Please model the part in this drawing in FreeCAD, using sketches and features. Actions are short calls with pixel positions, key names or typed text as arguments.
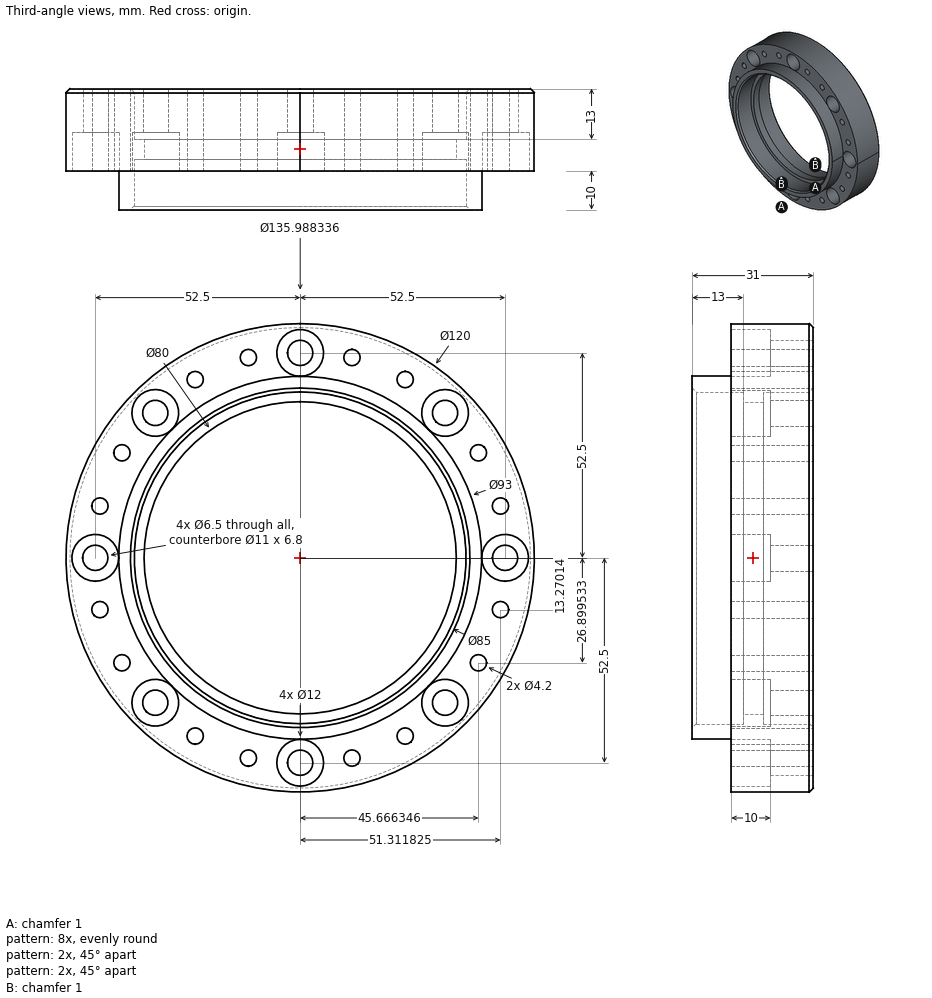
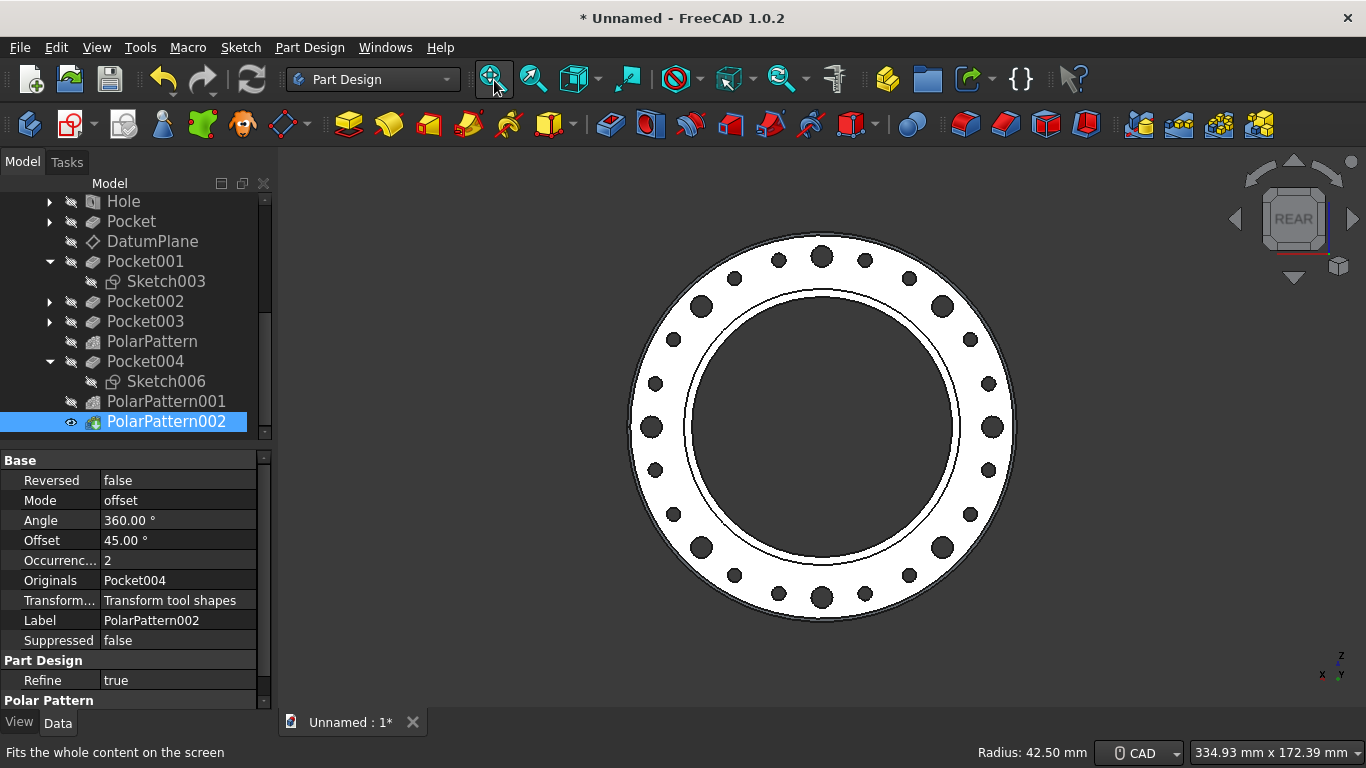
click(960, 426, ctrl)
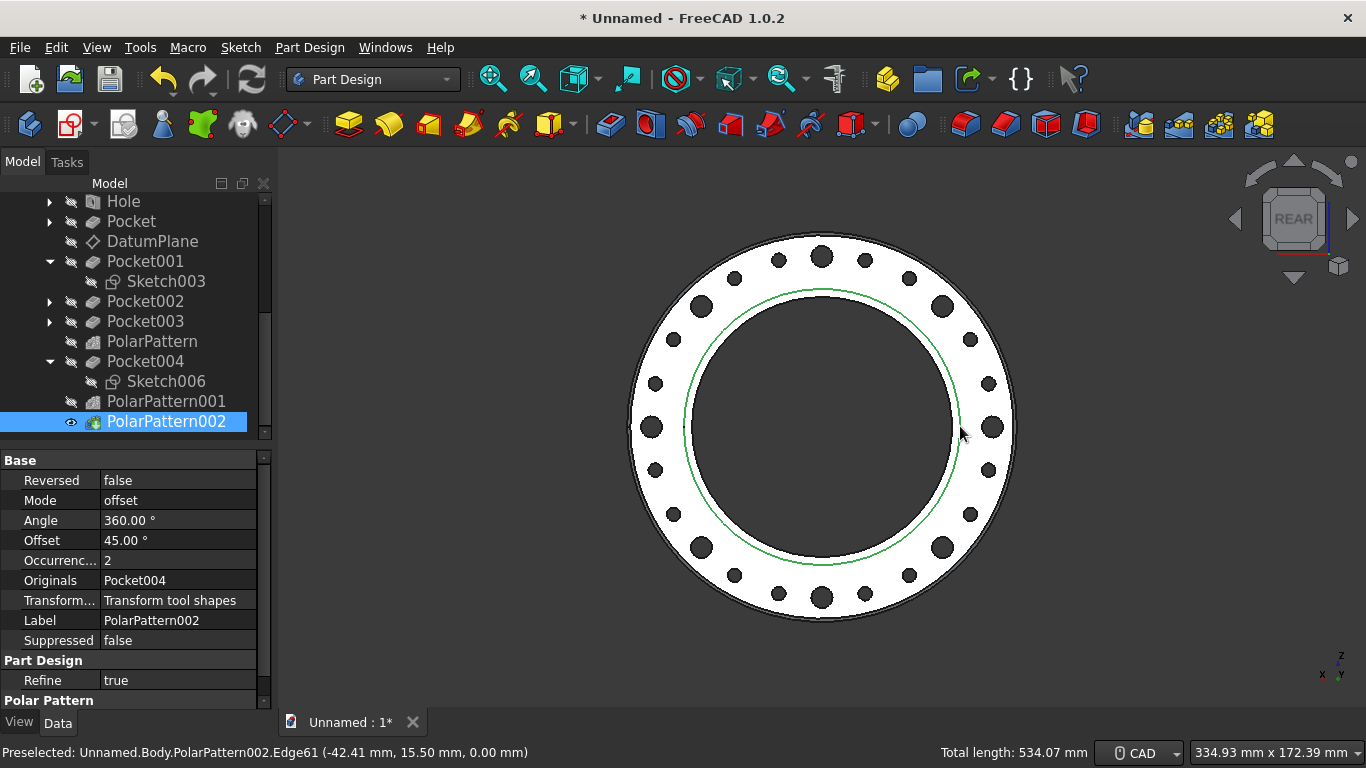
click(1006, 124)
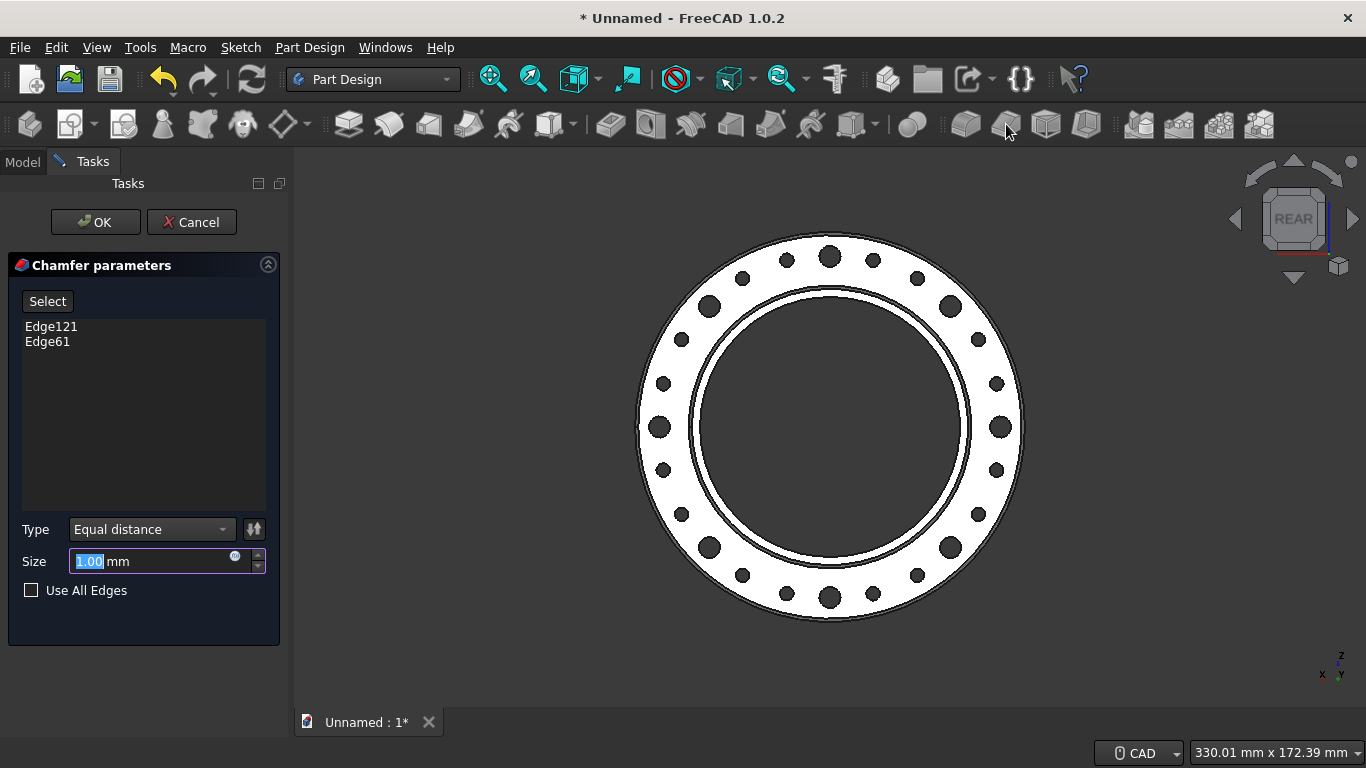
text(1)
key(Tab)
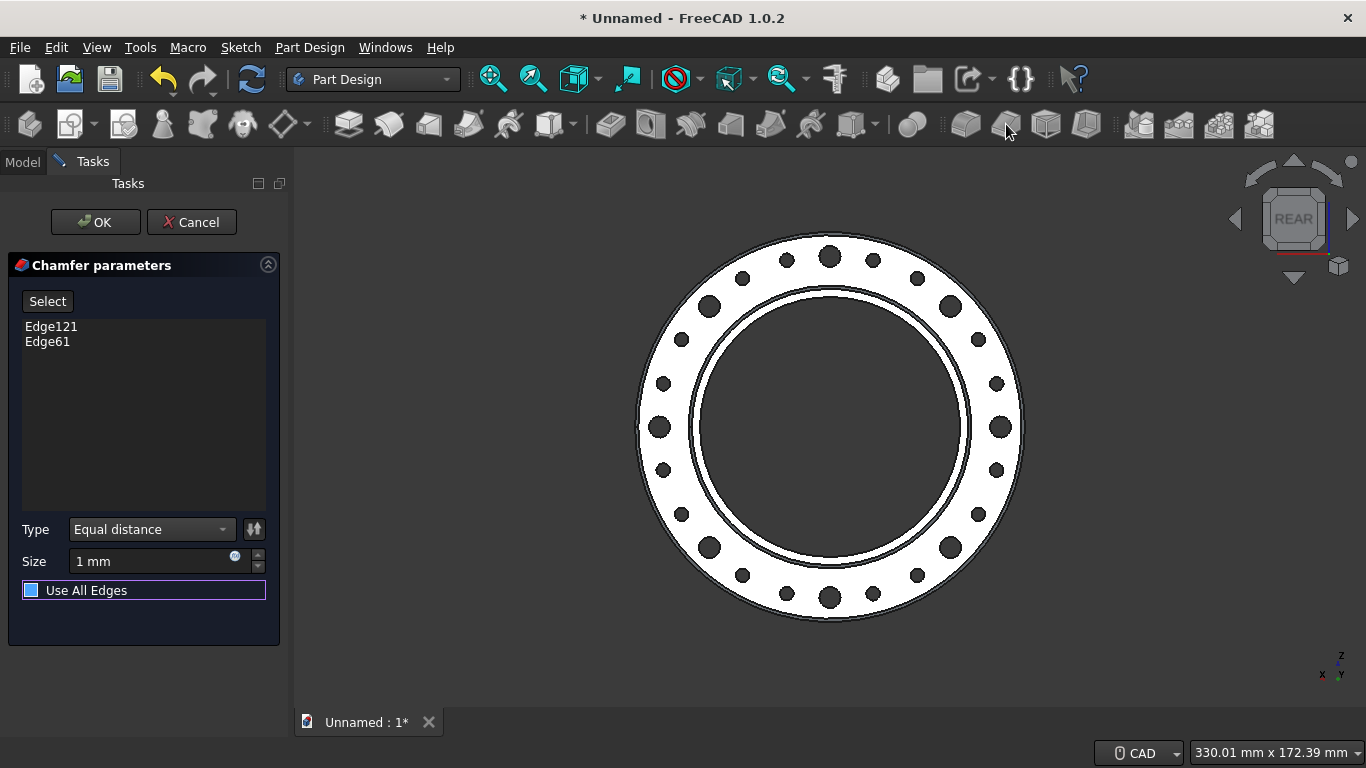
click(96, 222)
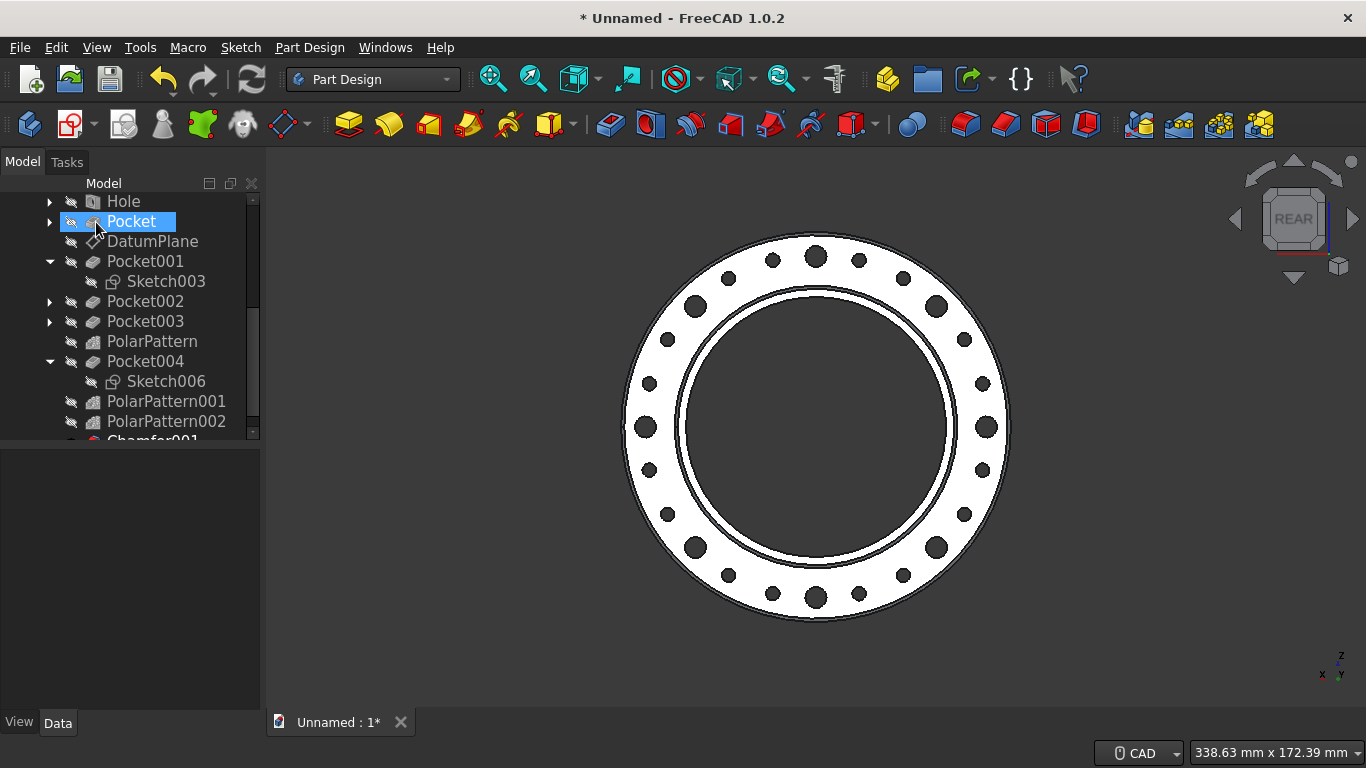
key(0)